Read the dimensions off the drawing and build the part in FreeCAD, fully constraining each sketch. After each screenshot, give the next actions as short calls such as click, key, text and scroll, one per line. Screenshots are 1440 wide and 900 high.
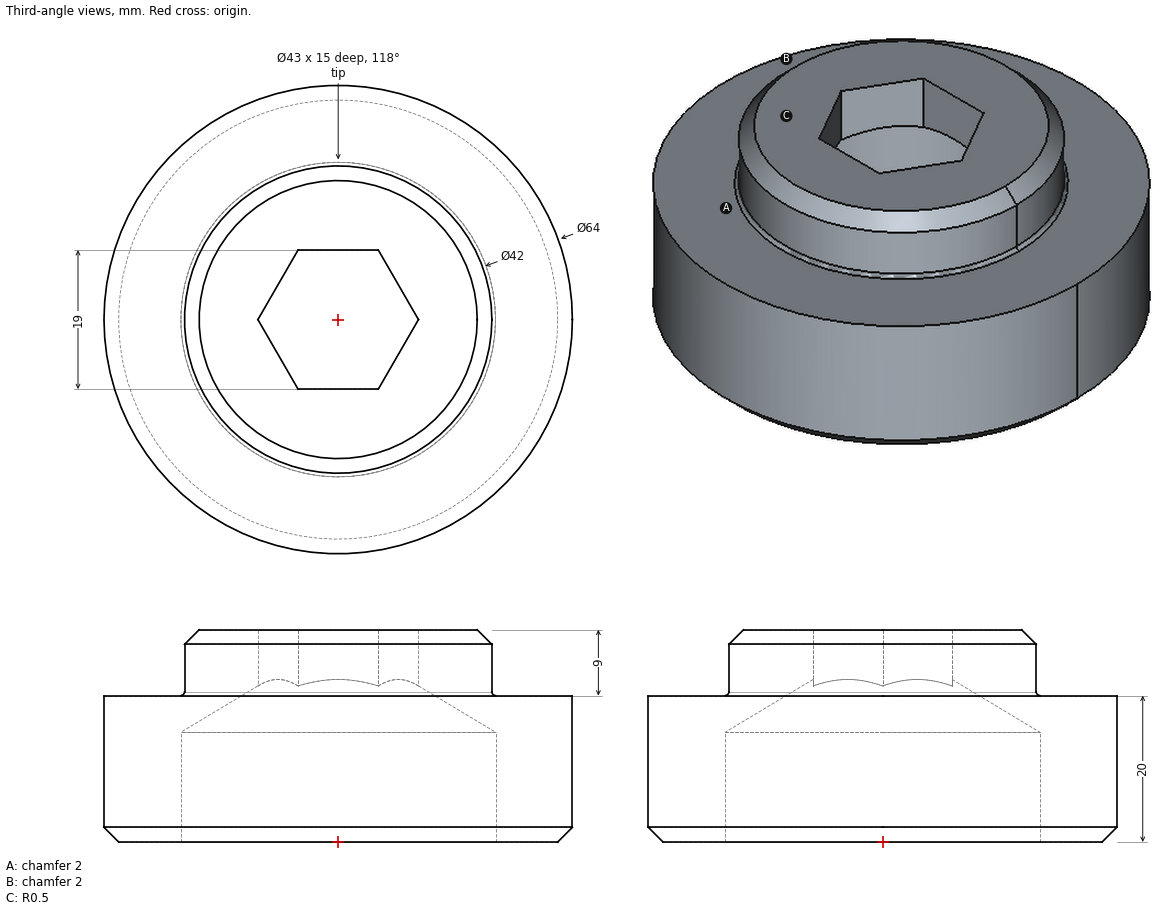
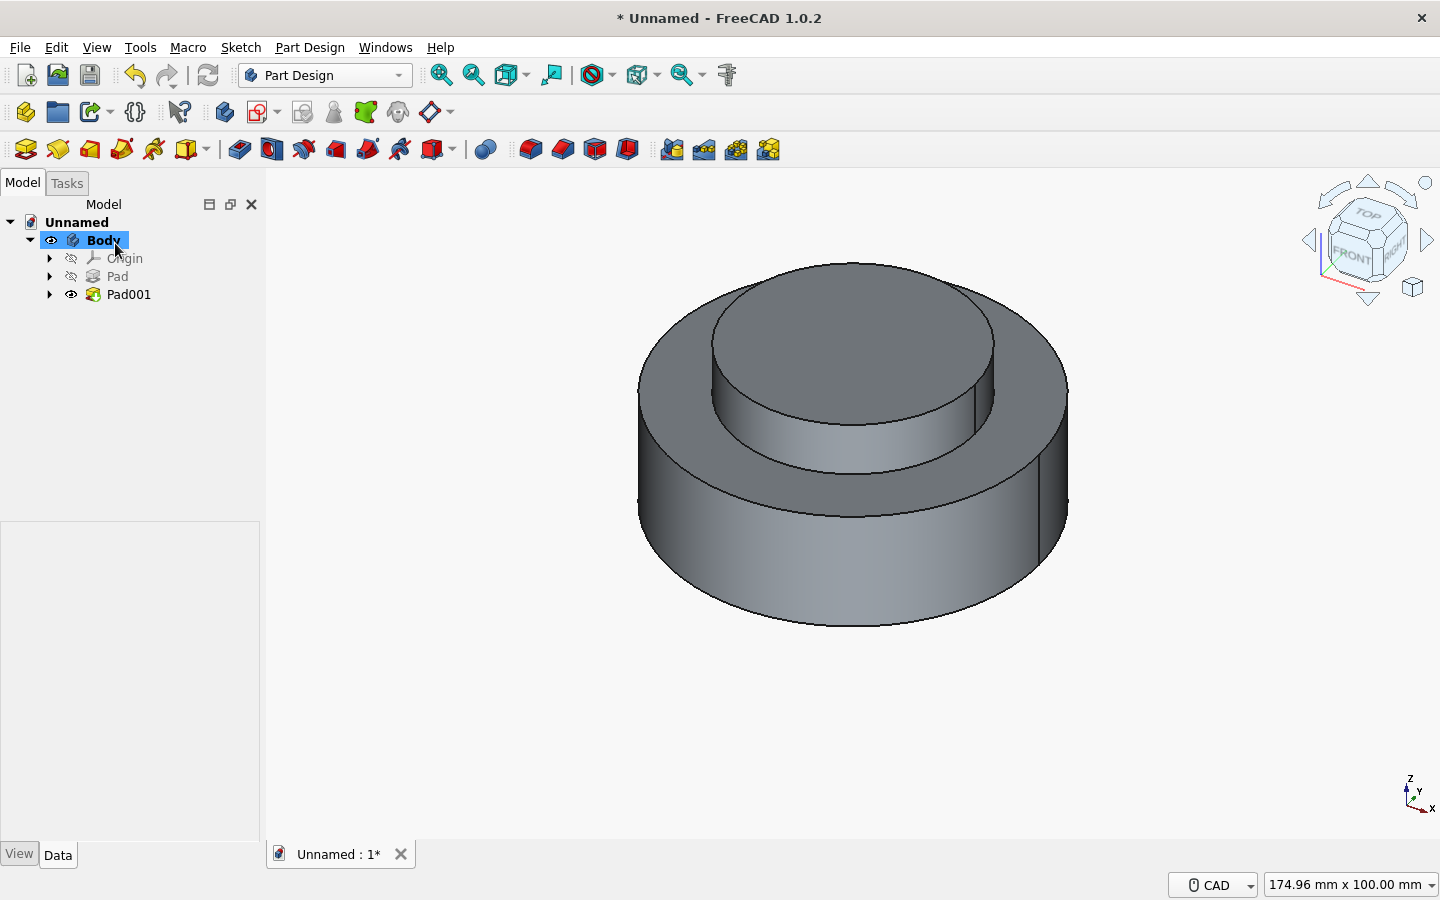
key(5)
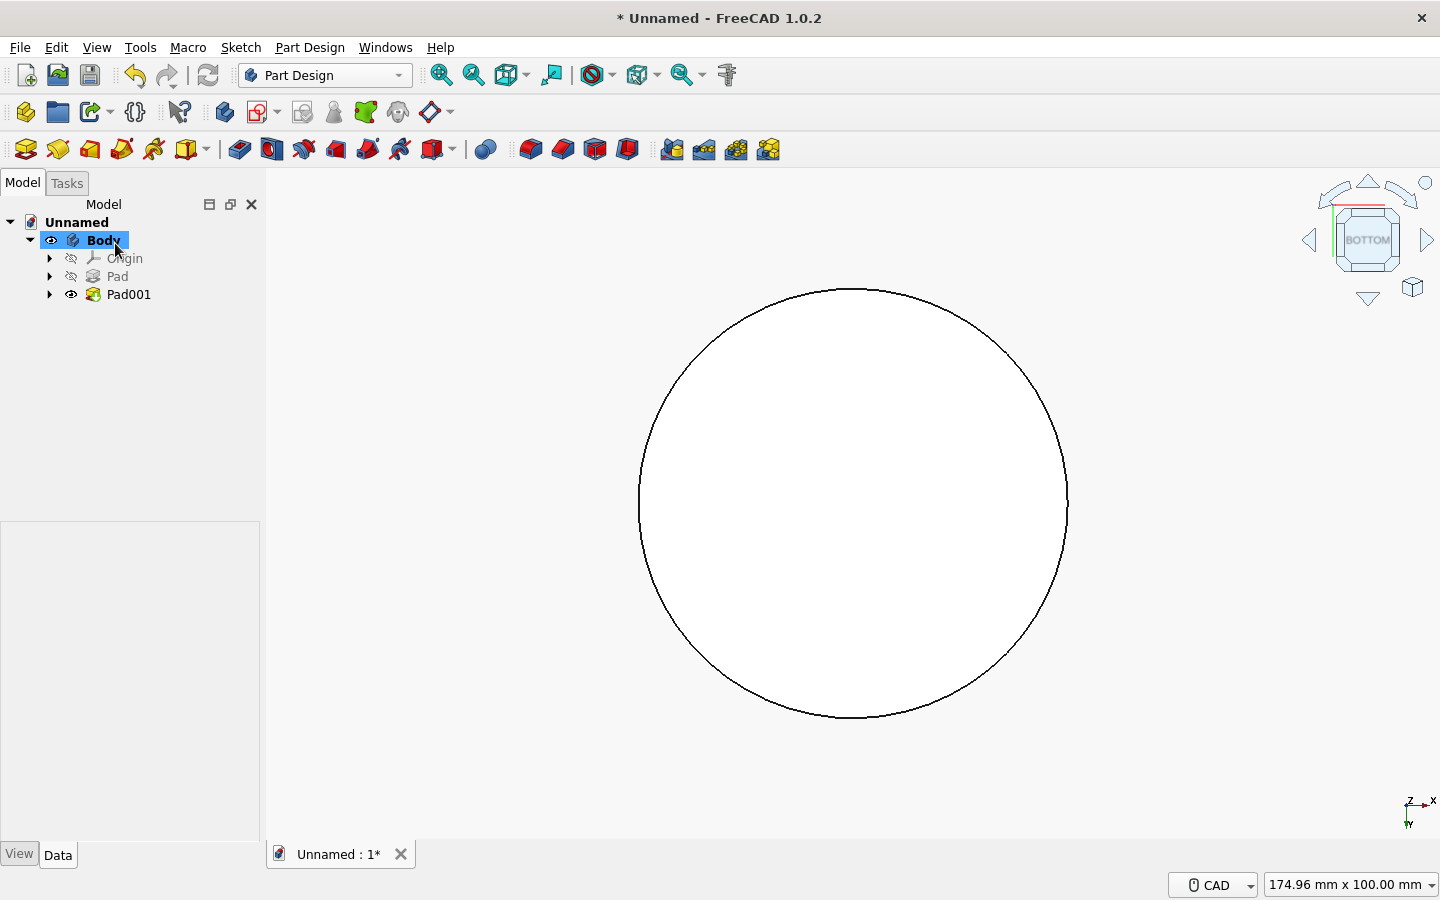
click(853, 502)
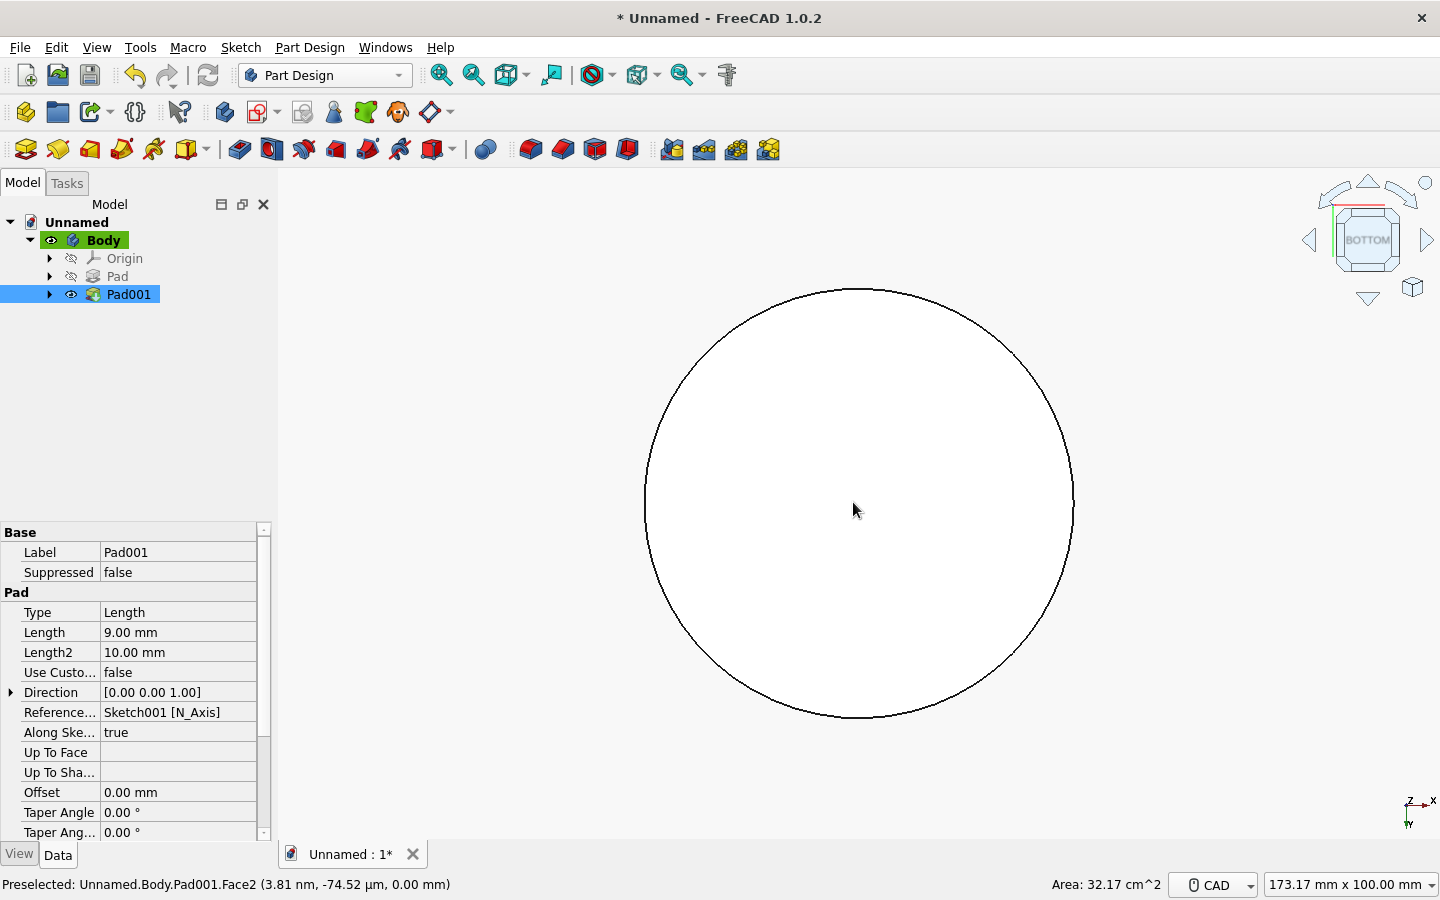
click(258, 112)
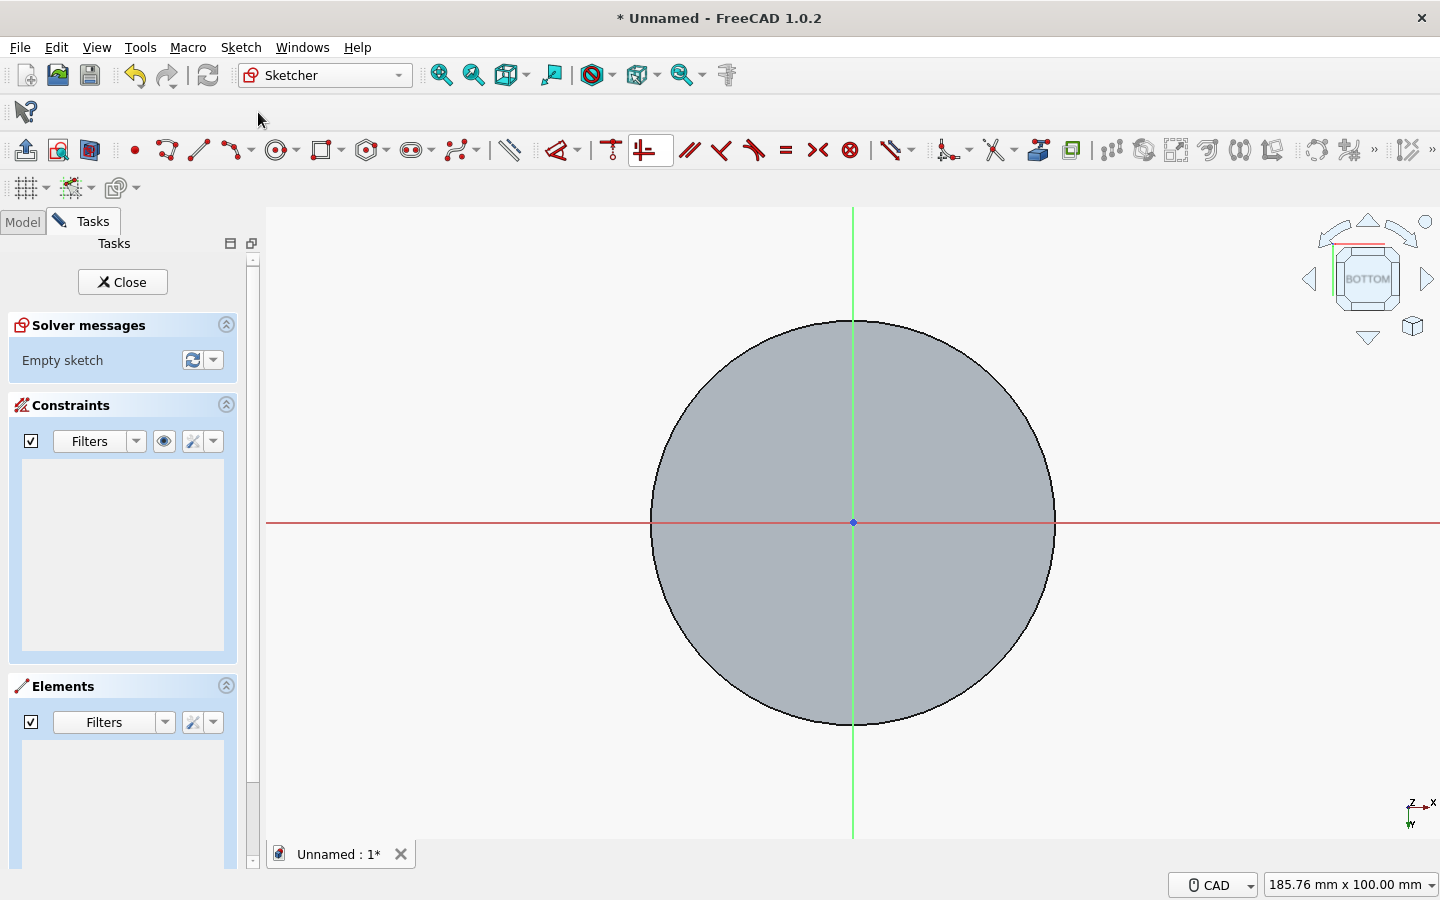
scroll(992, 523, up, 2)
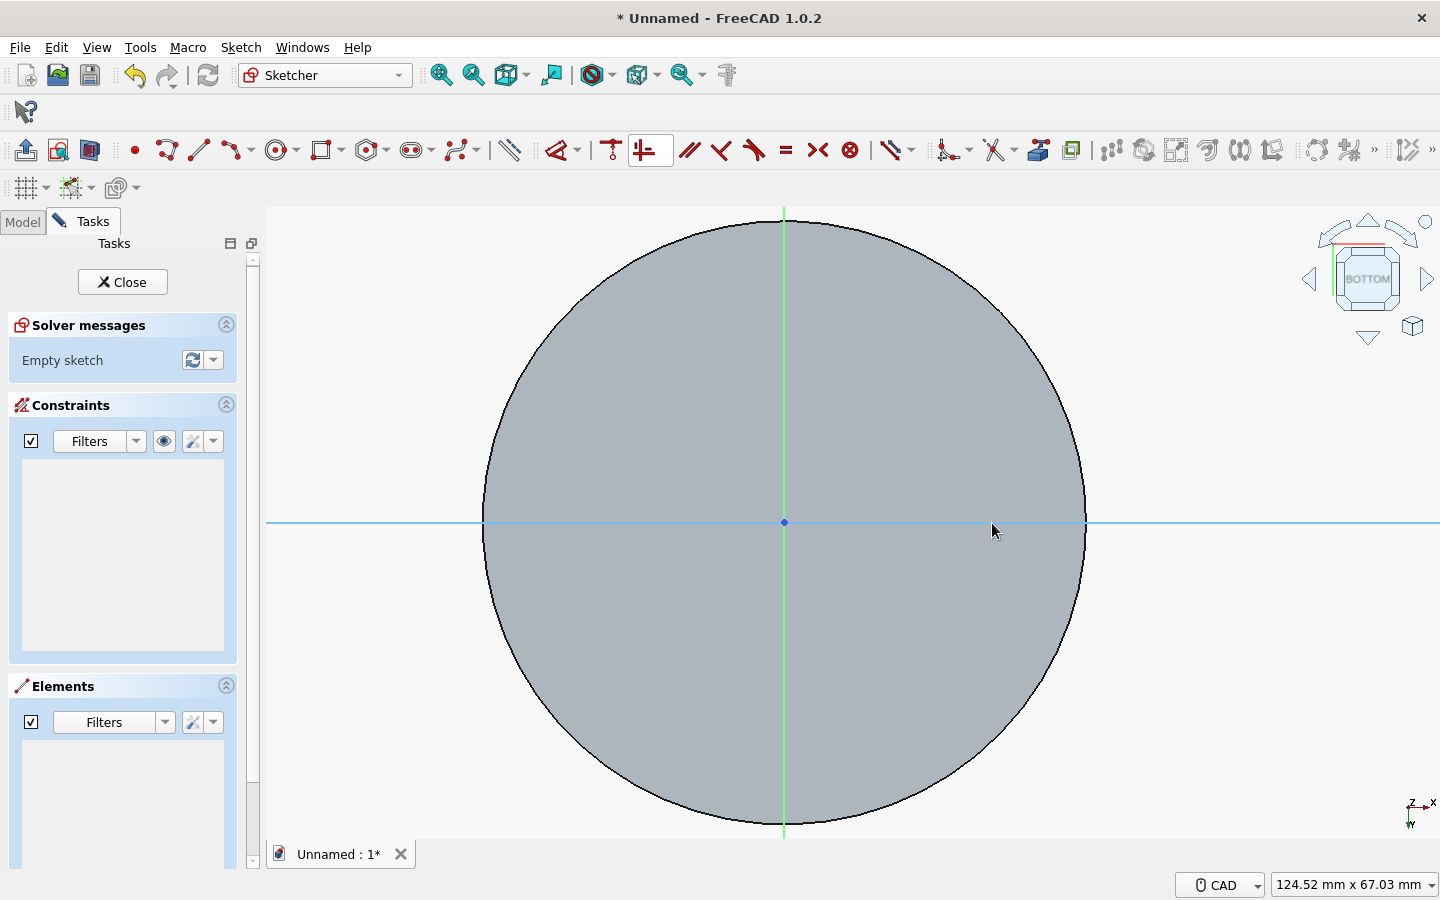
click(276, 150)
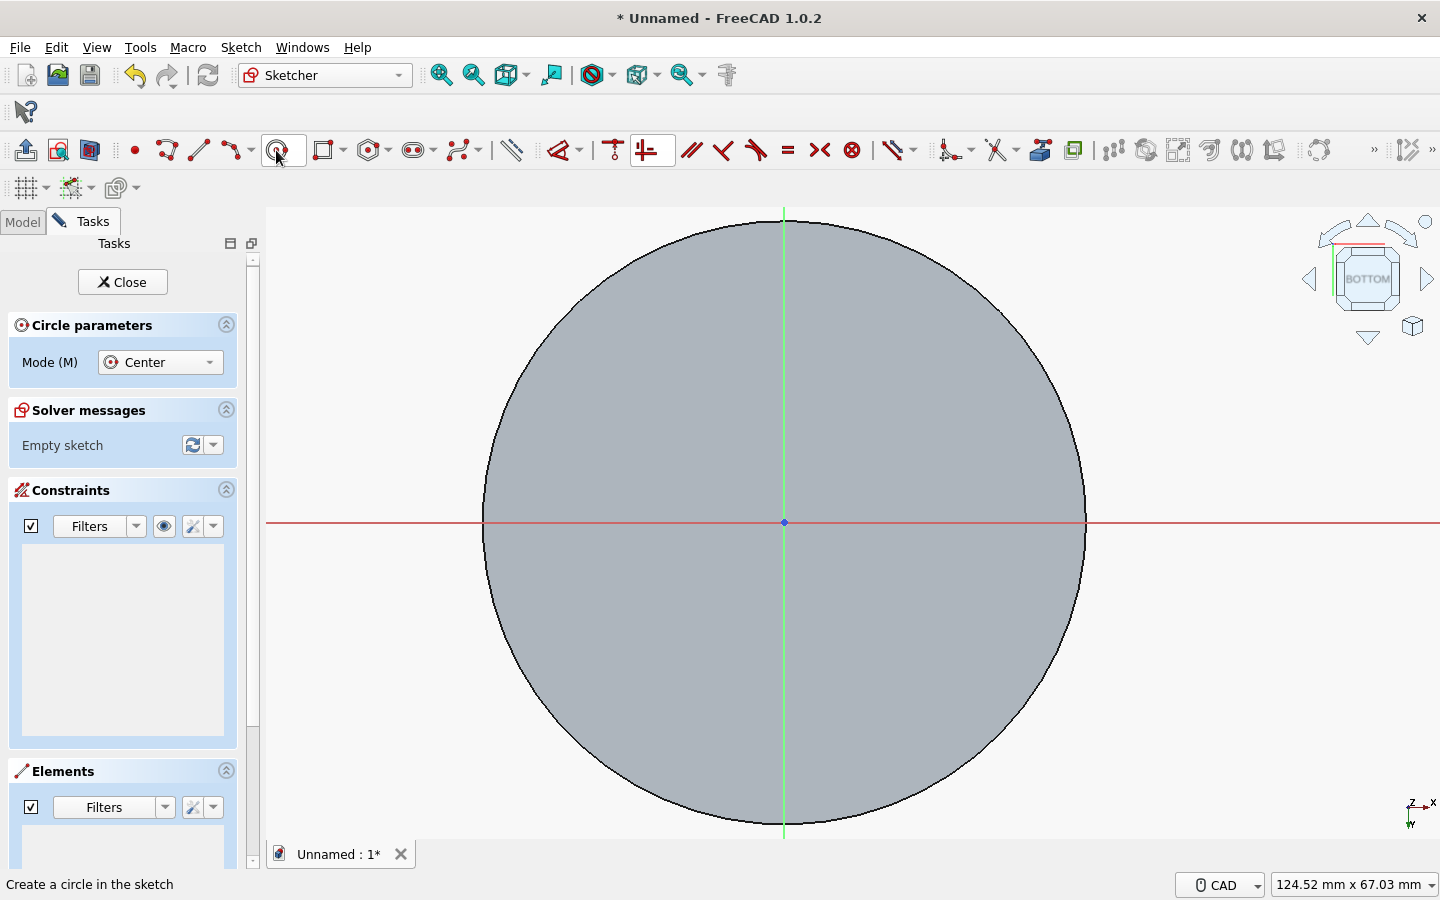
click(784, 523)
move(928, 379)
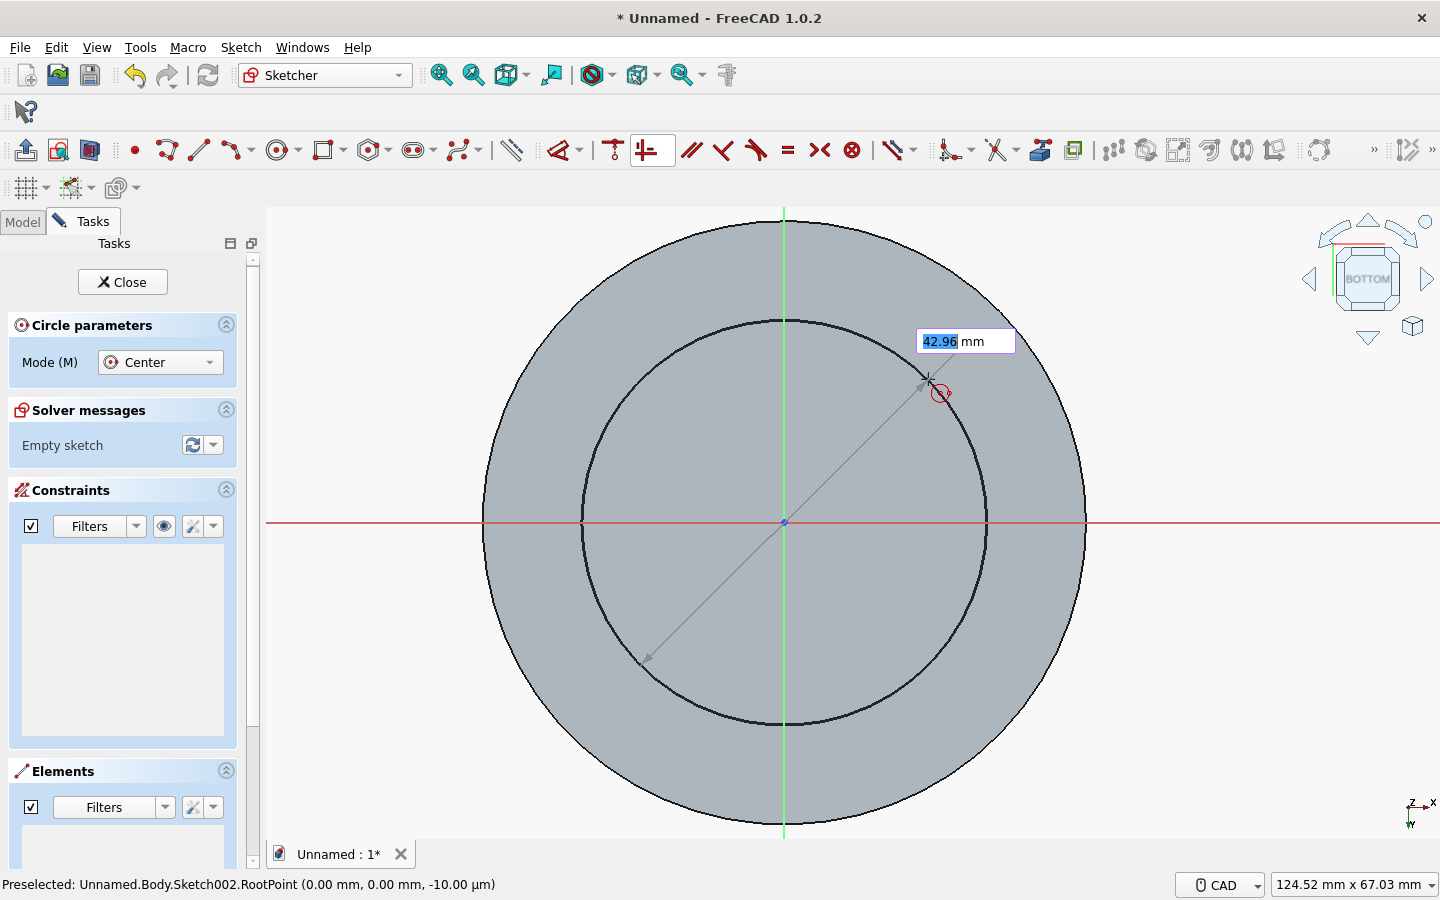
text(43)
key(Return)
key(Escape)